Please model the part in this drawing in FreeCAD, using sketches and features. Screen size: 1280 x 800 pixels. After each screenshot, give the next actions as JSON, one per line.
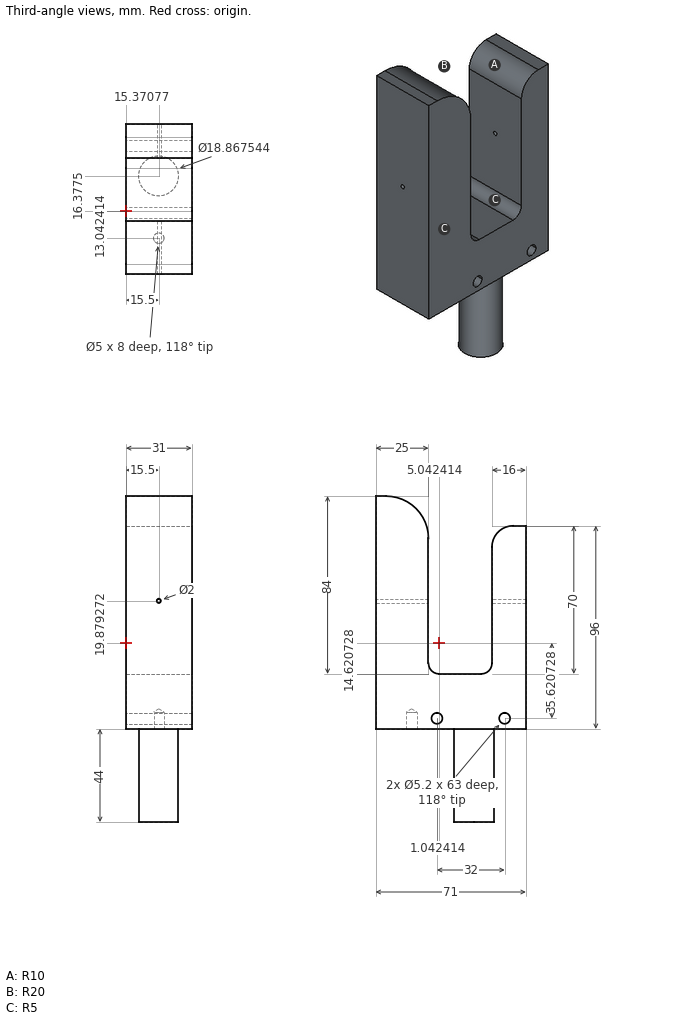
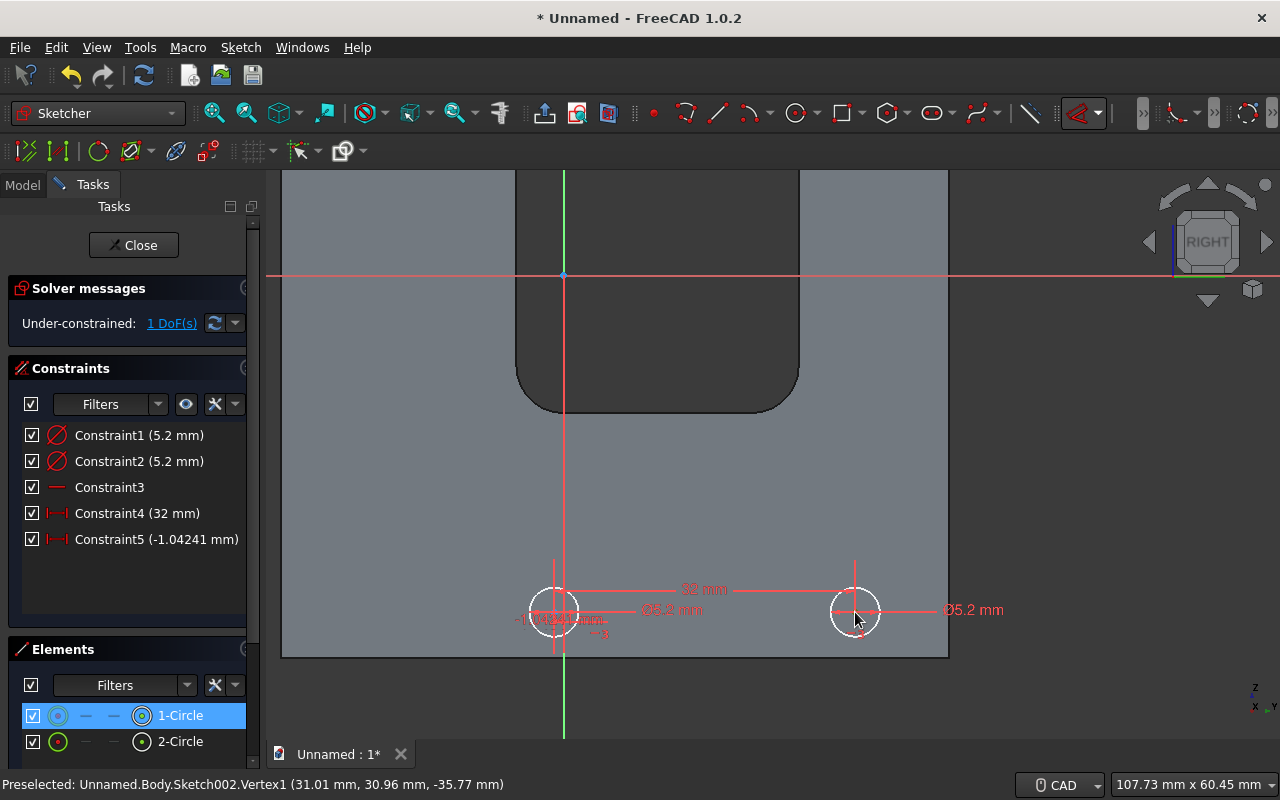
{"action": "key", "text": "i"}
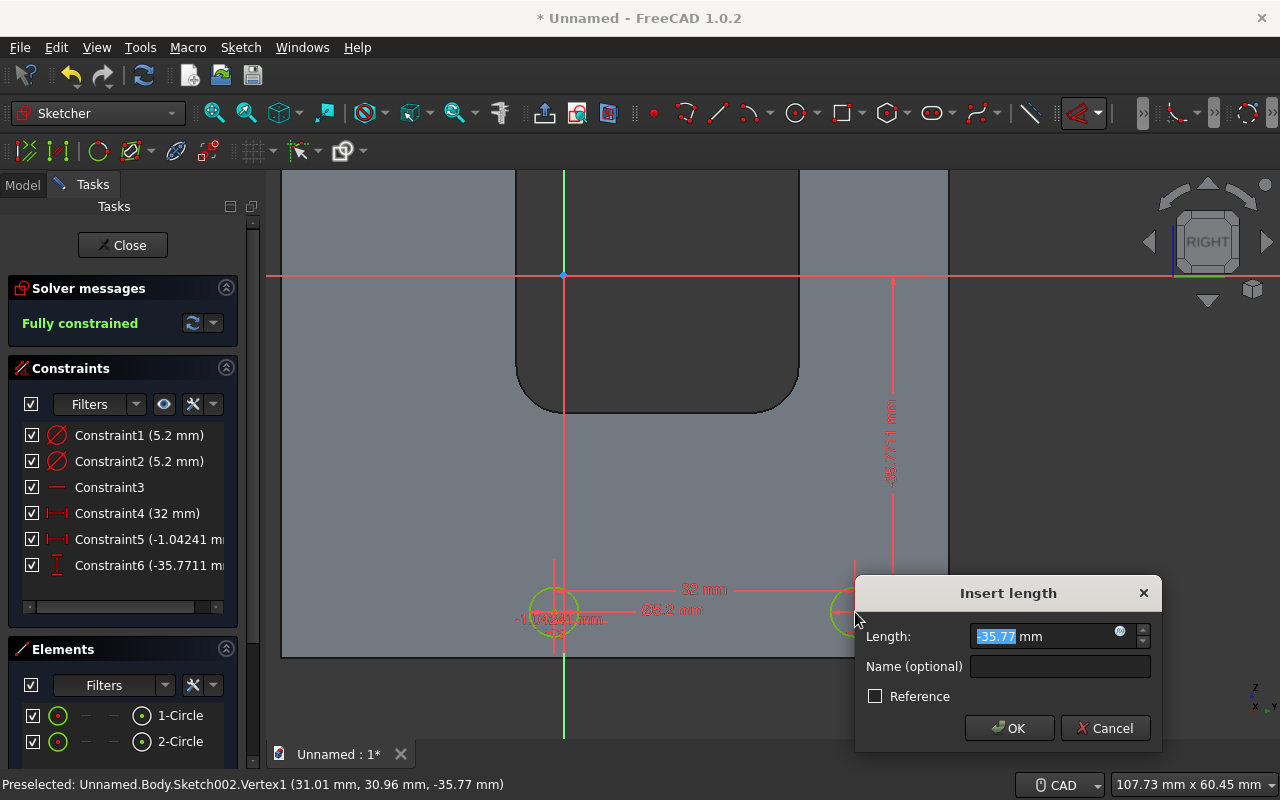
{"action": "type", "text": "-35.620728"}
{"action": "key", "text": "Return"}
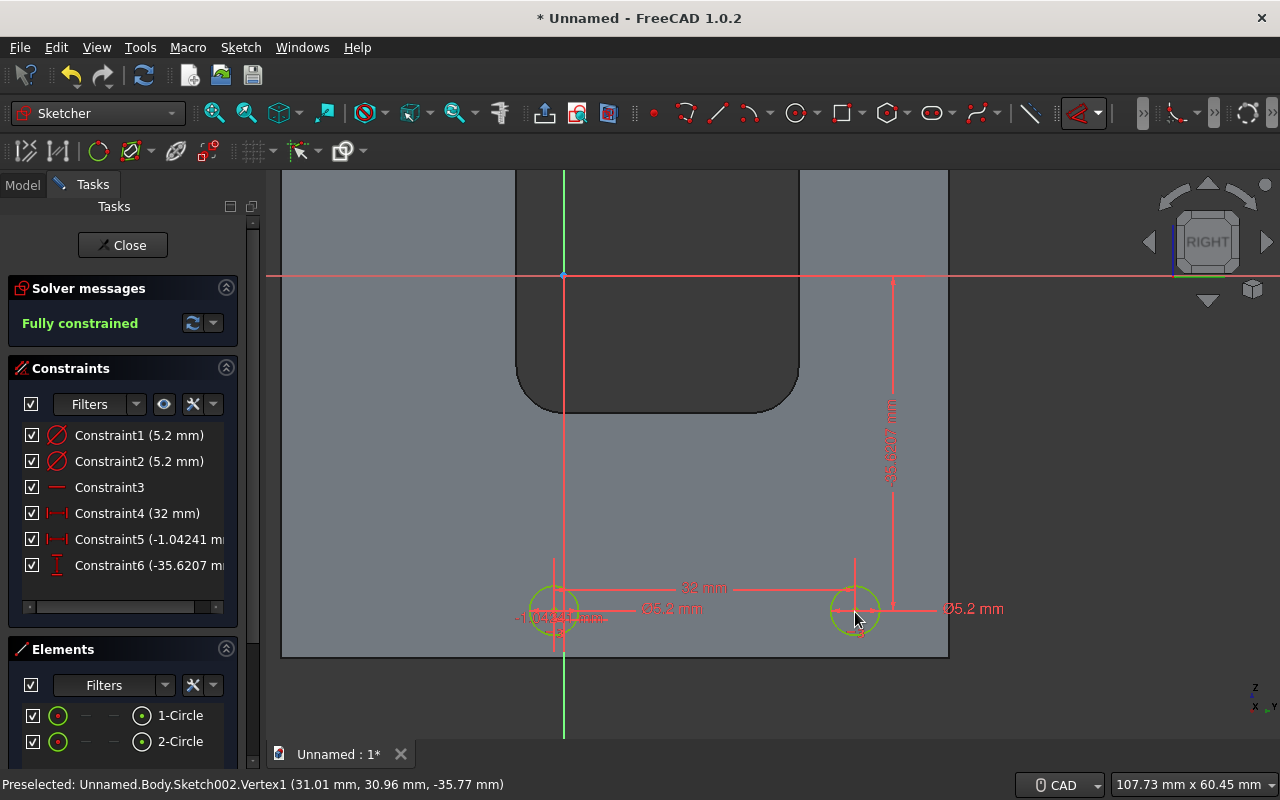
{"action": "left_click", "coordinate": [123, 245]}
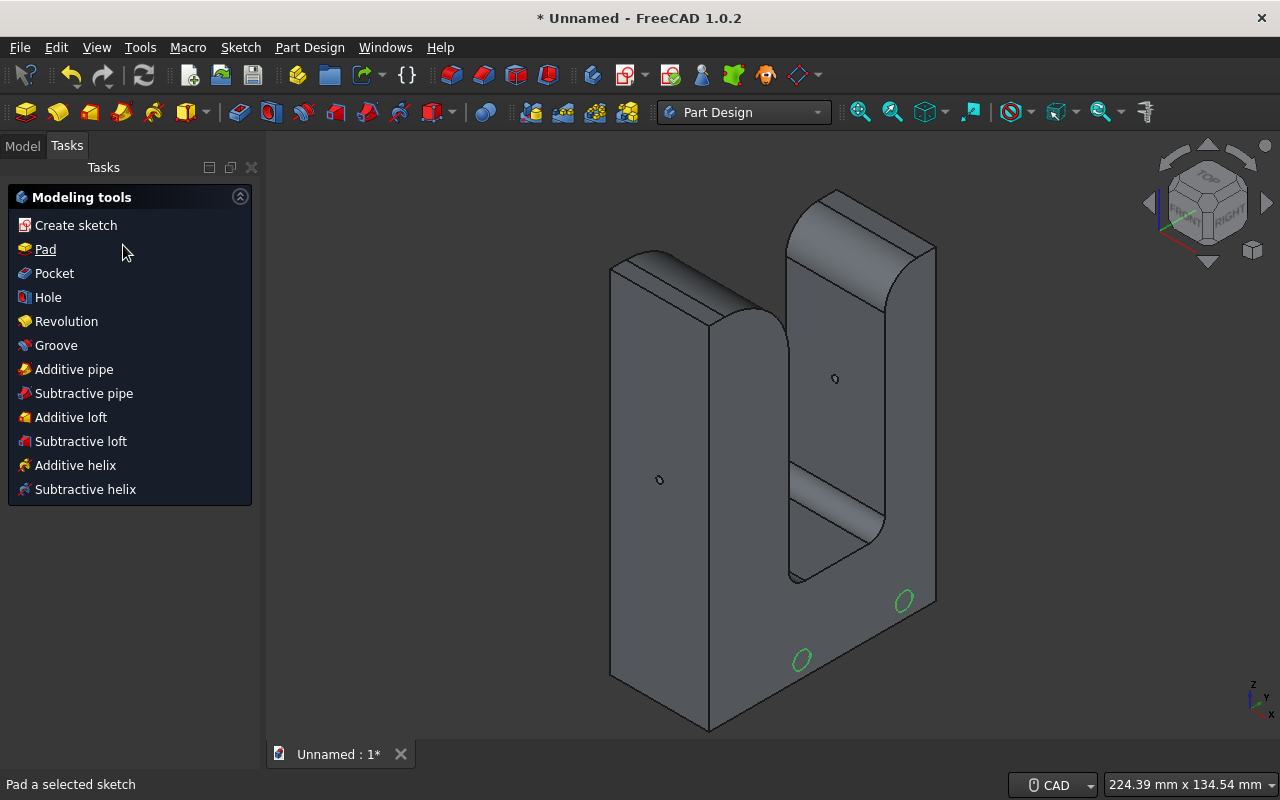
{"action": "left_click", "coordinate": [272, 112]}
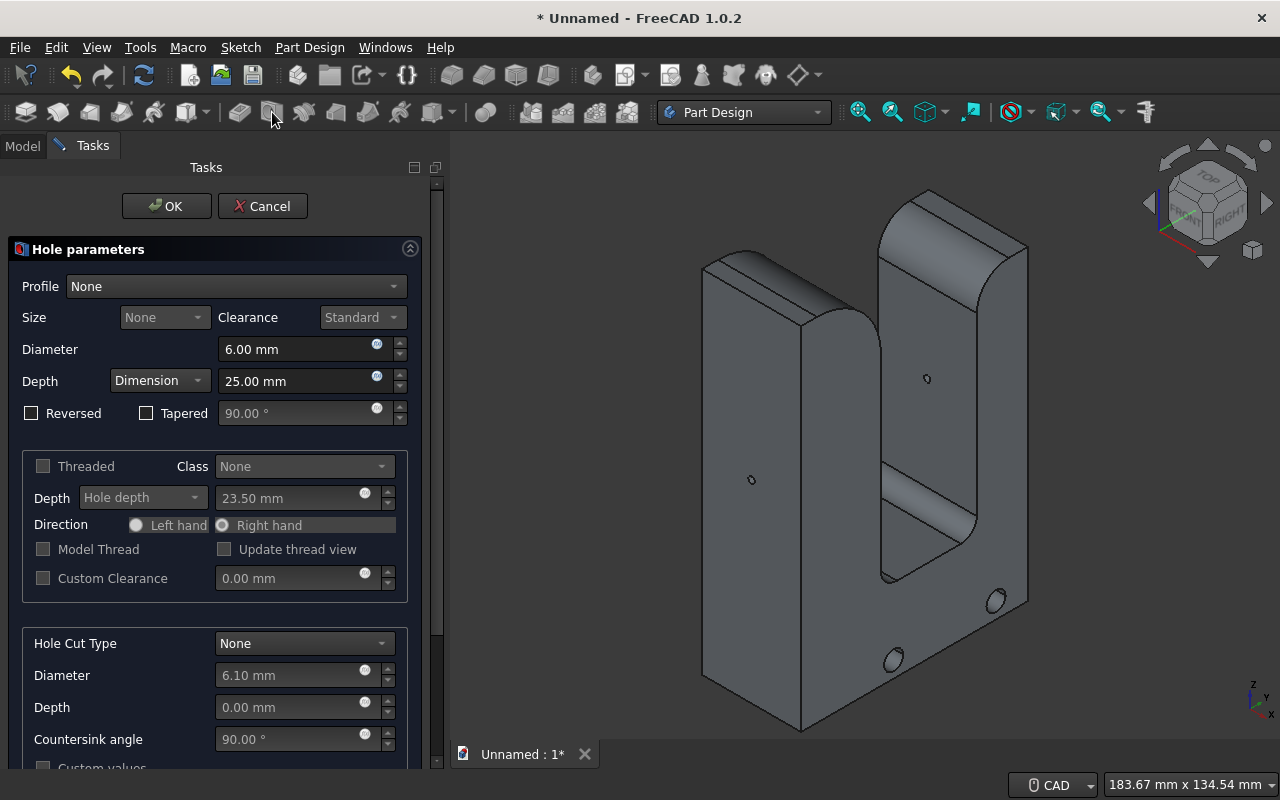
{"action": "triple_click", "coordinate": [305, 349]}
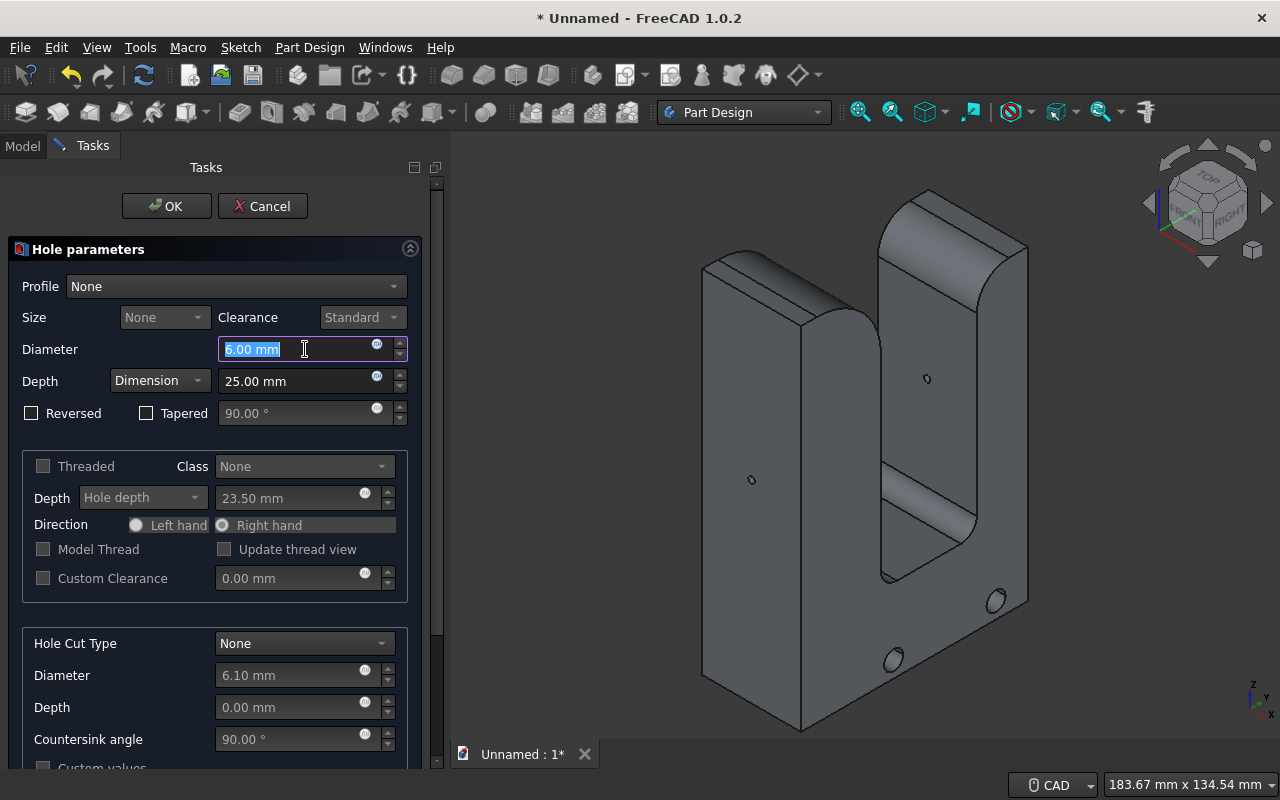
{"action": "type", "text": "5.2"}
{"action": "key", "text": "Tab"}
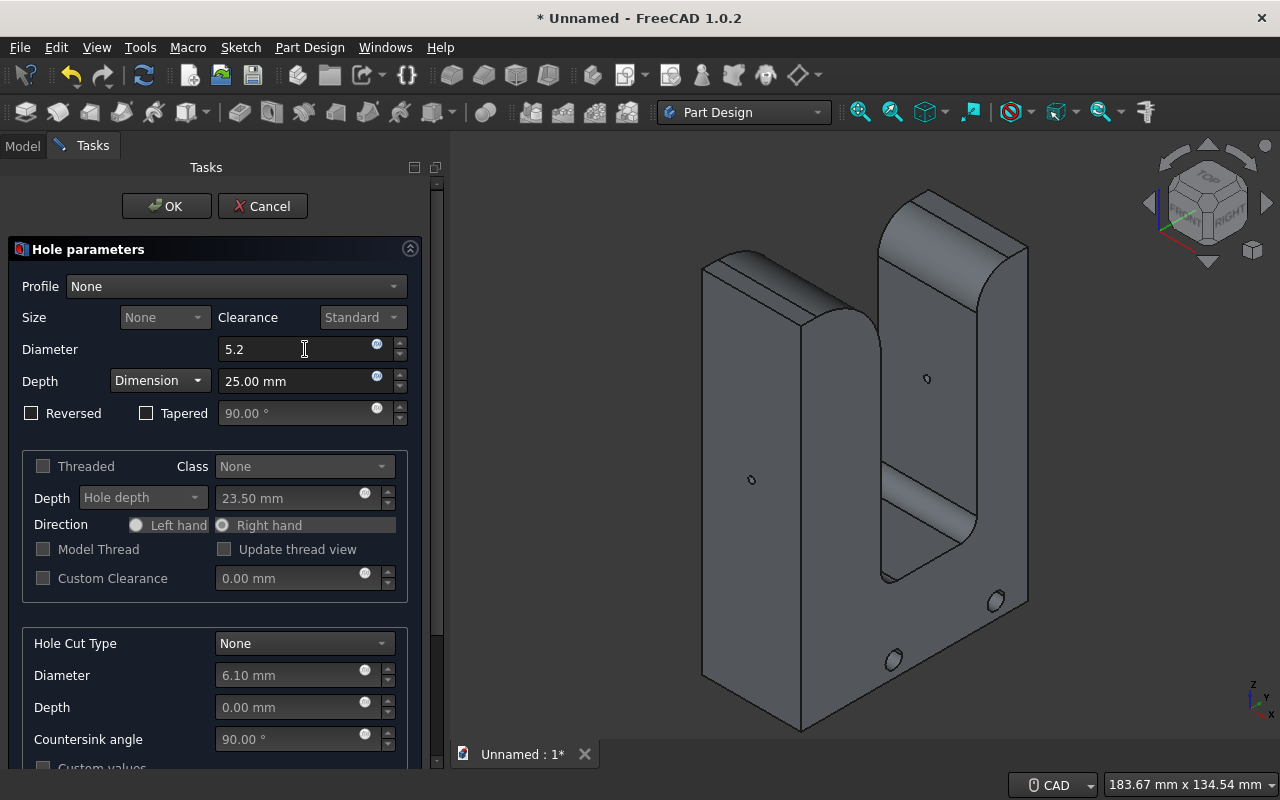
{"action": "triple_click", "coordinate": [305, 381]}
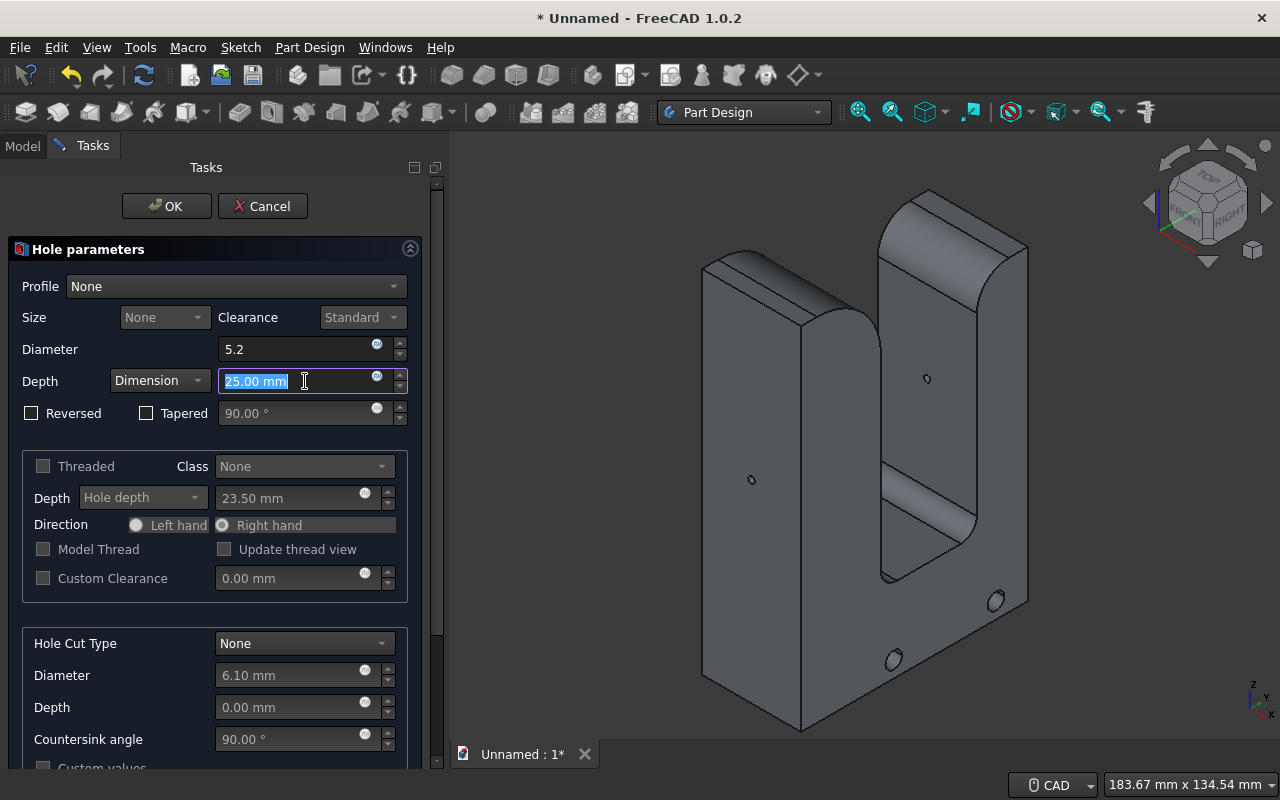
{"action": "type", "text": "63"}
{"action": "key", "text": "Tab"}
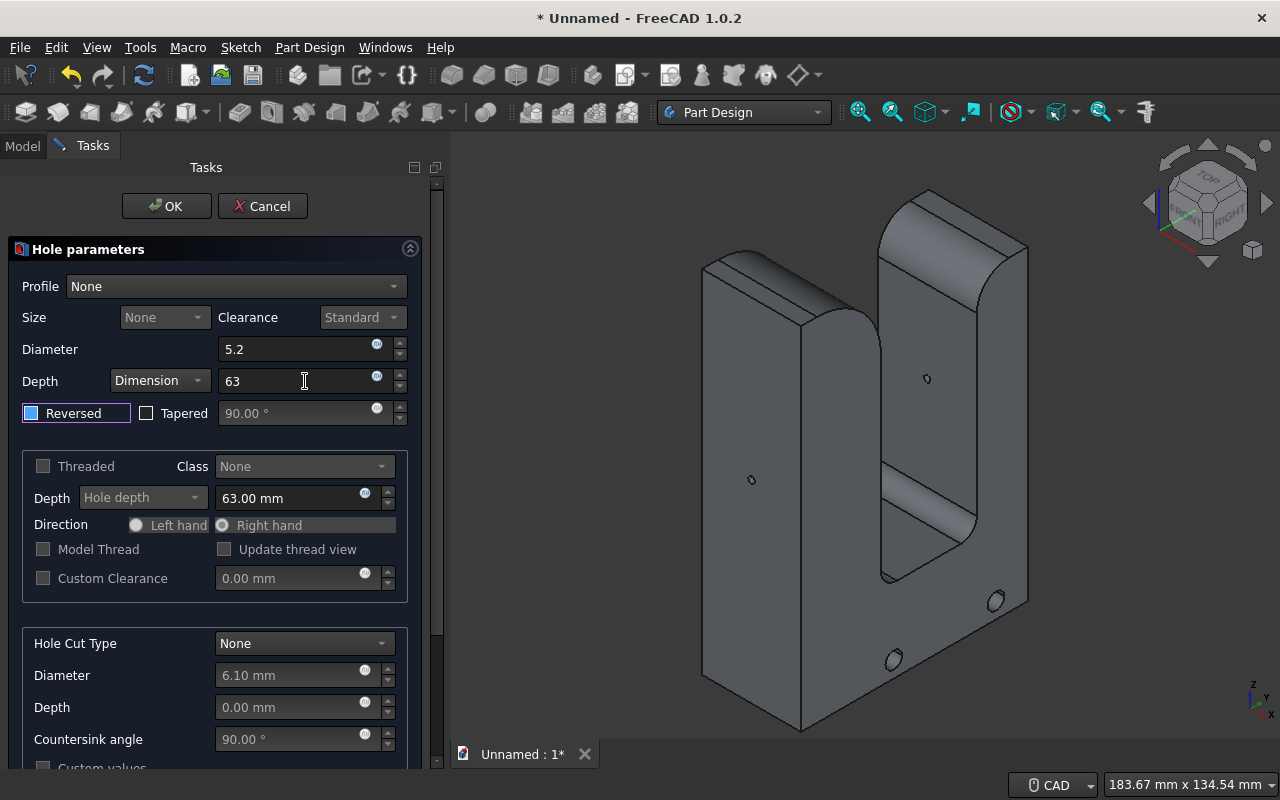
{"action": "left_click", "coordinate": [167, 206]}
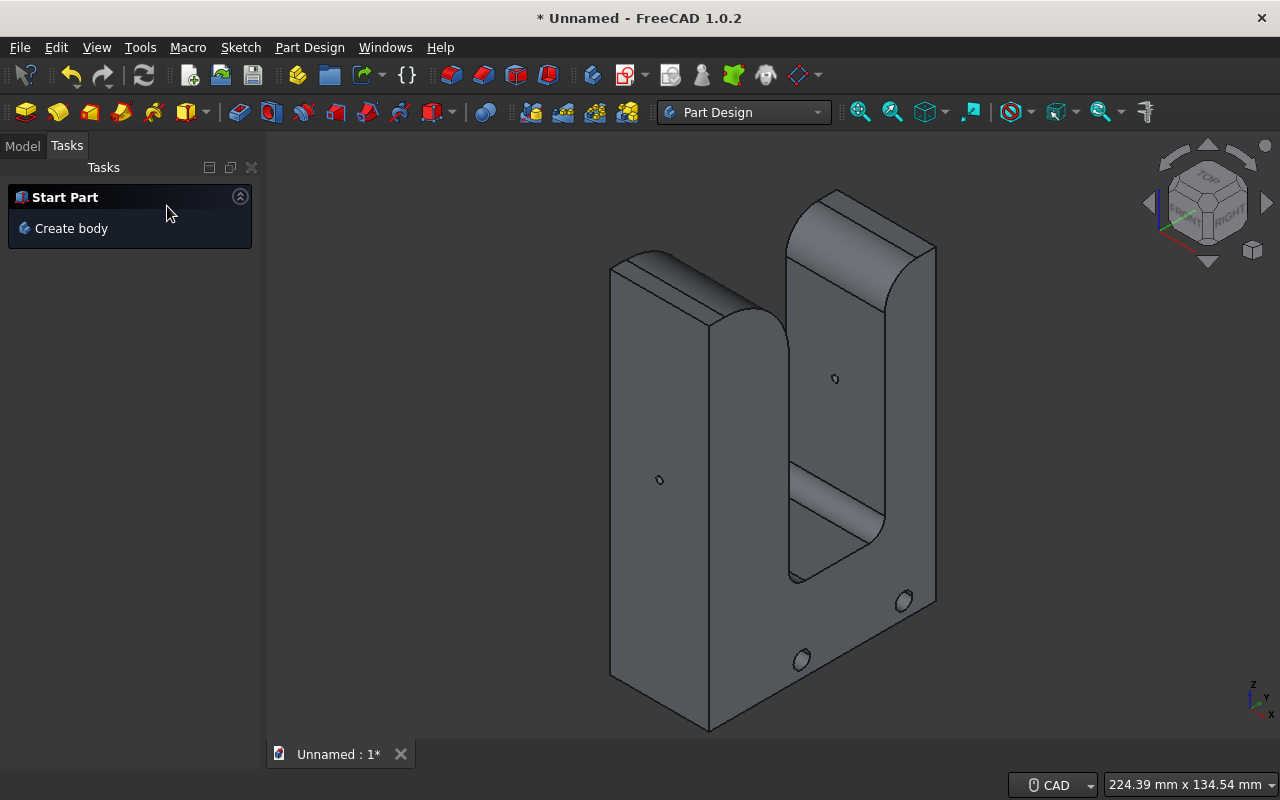
{"action": "key", "text": "5"}